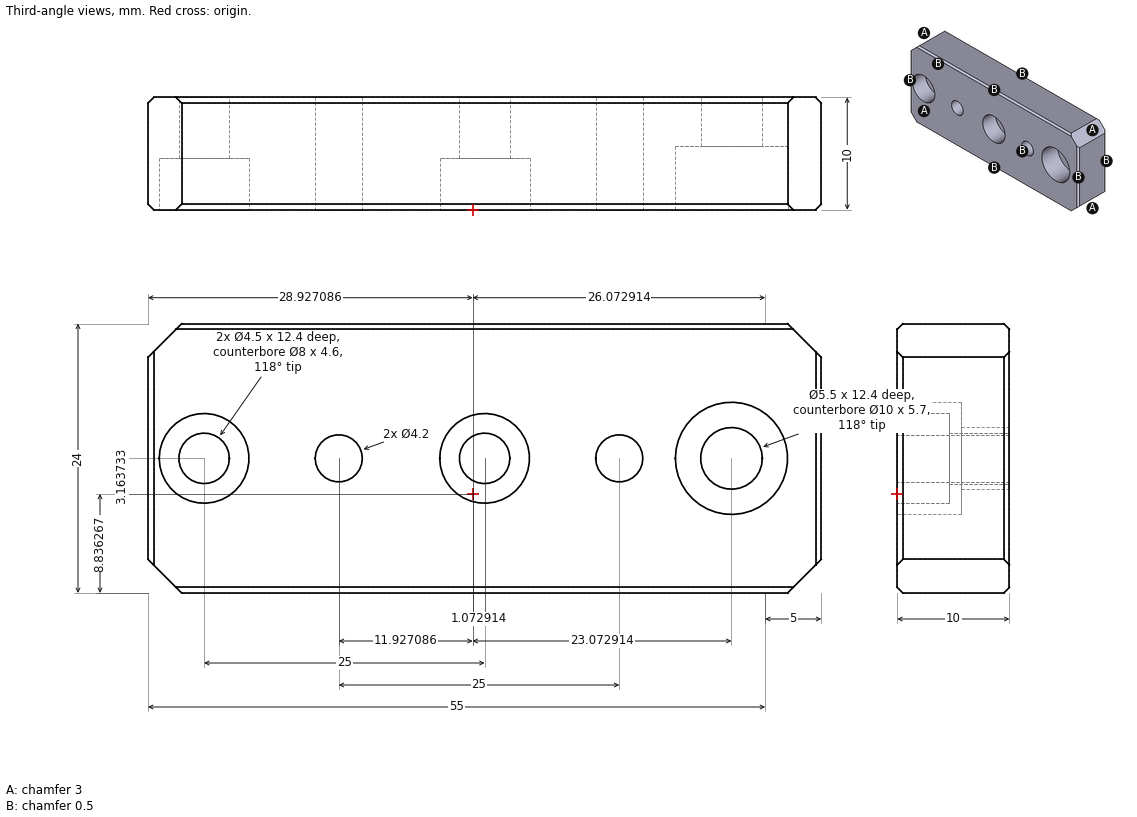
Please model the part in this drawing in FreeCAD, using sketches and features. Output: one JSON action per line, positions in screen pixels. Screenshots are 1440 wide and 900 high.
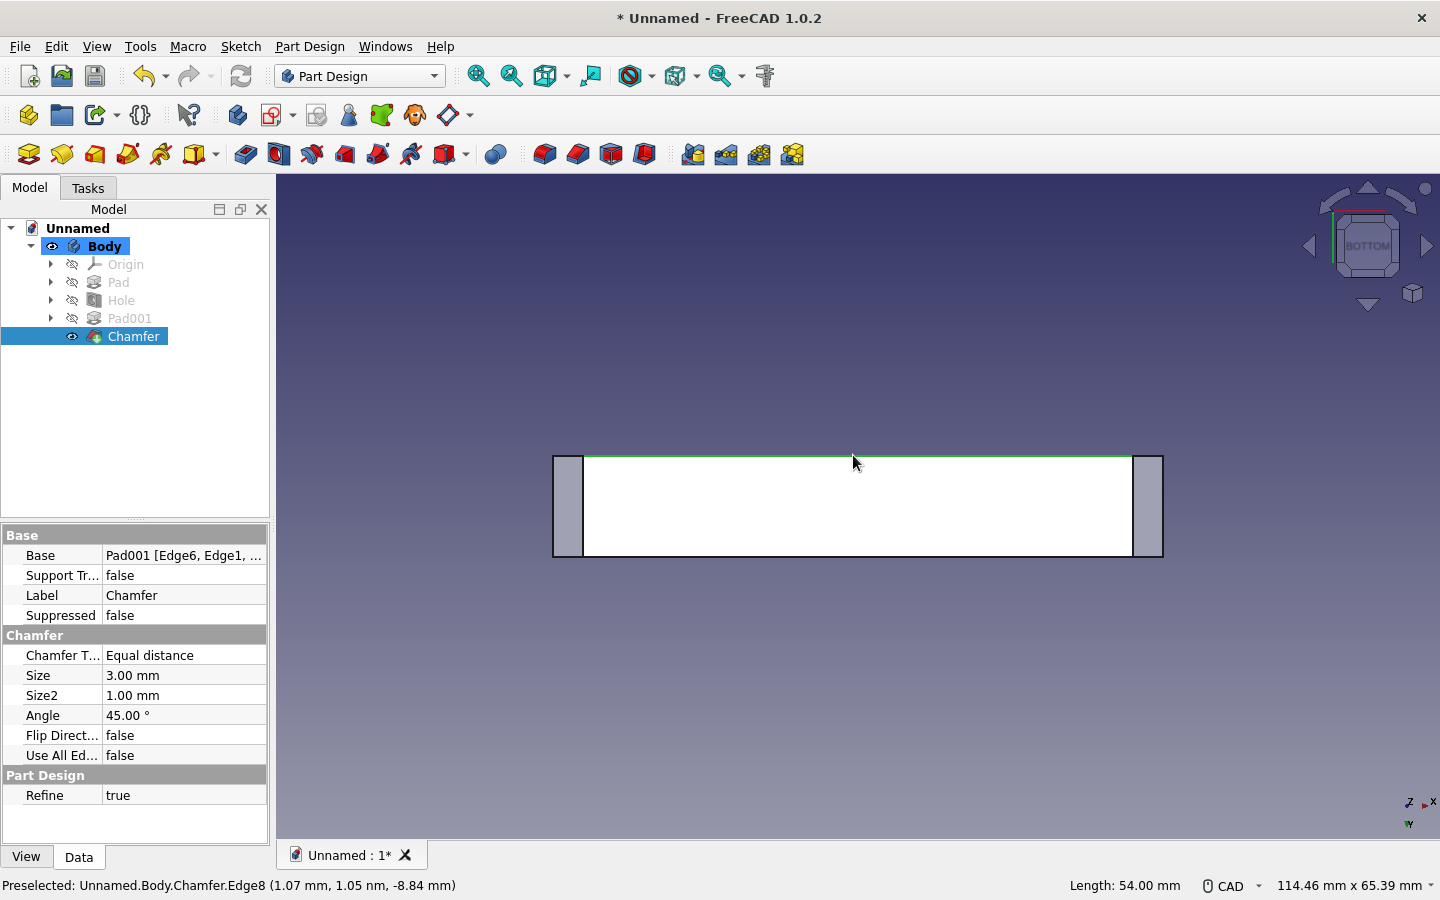
{"action": "key", "text": "0"}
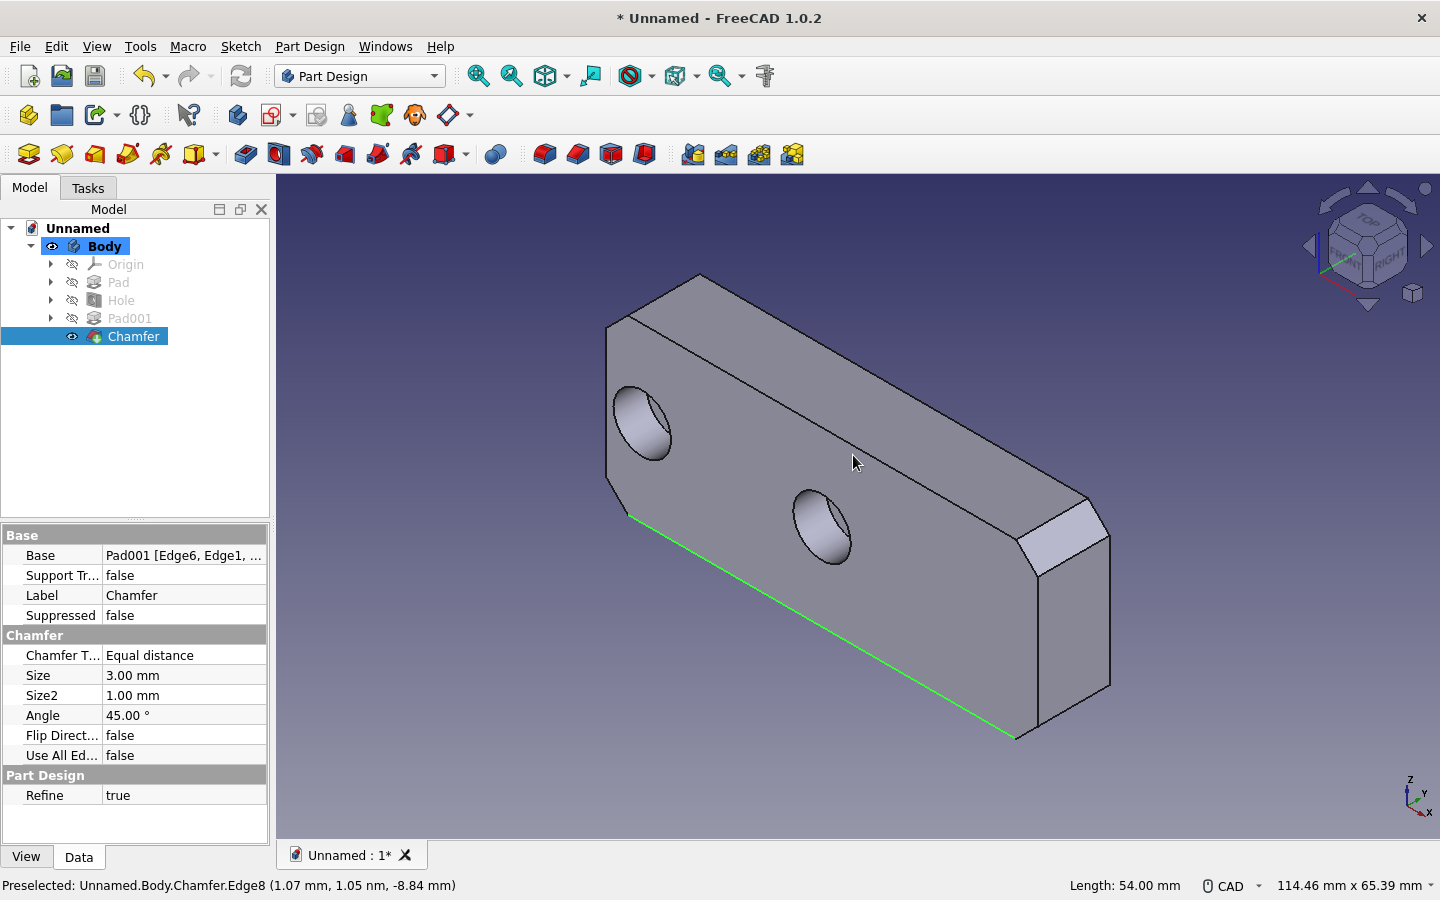
{"action": "left_click", "coordinate": [1038, 651], "text": "ctrl"}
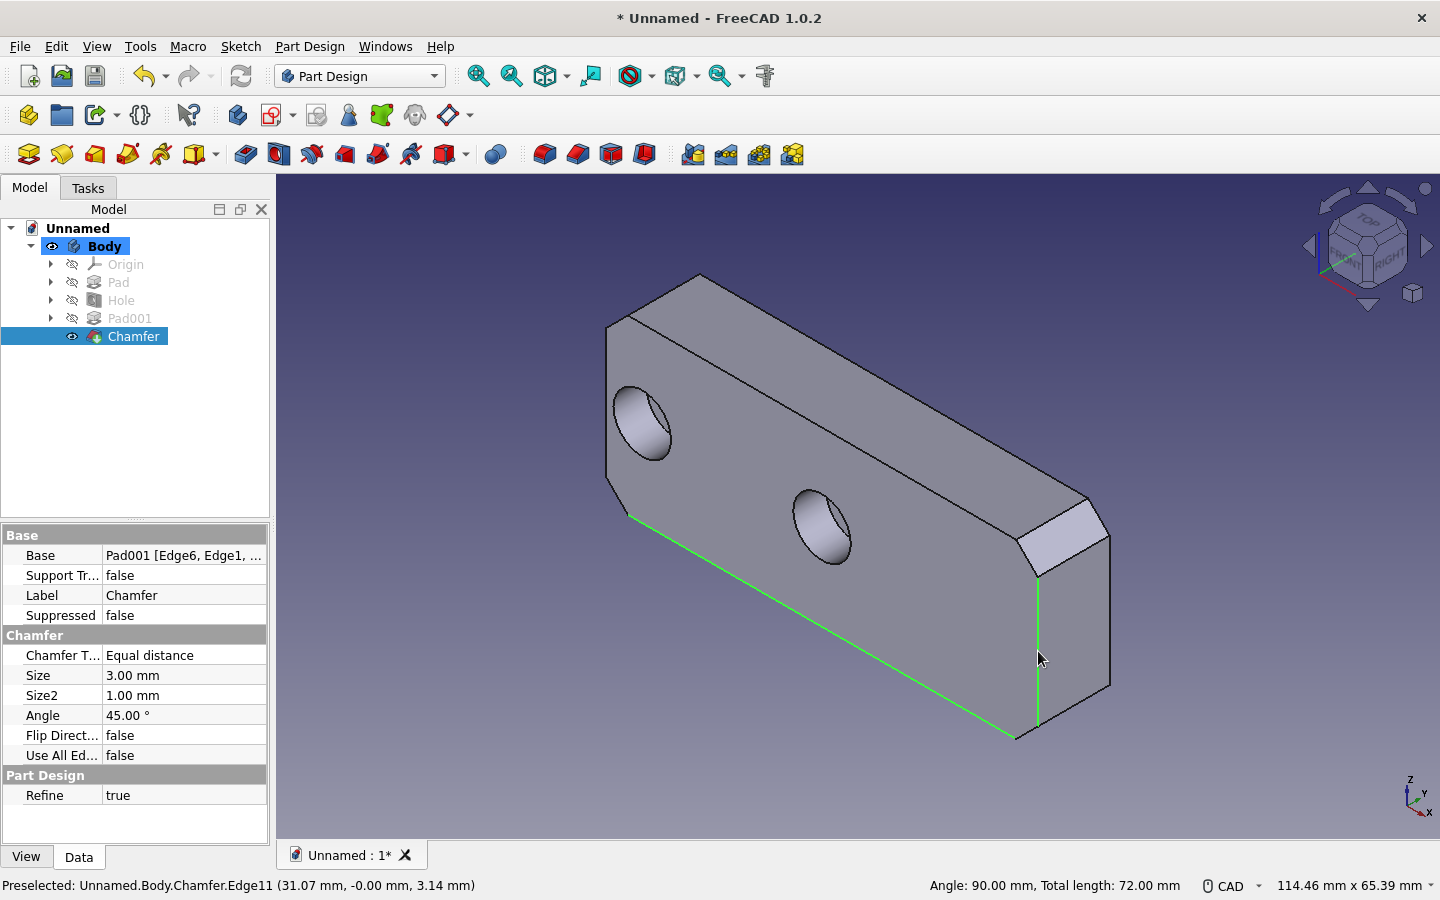
{"action": "left_click", "coordinate": [822, 427], "text": "ctrl"}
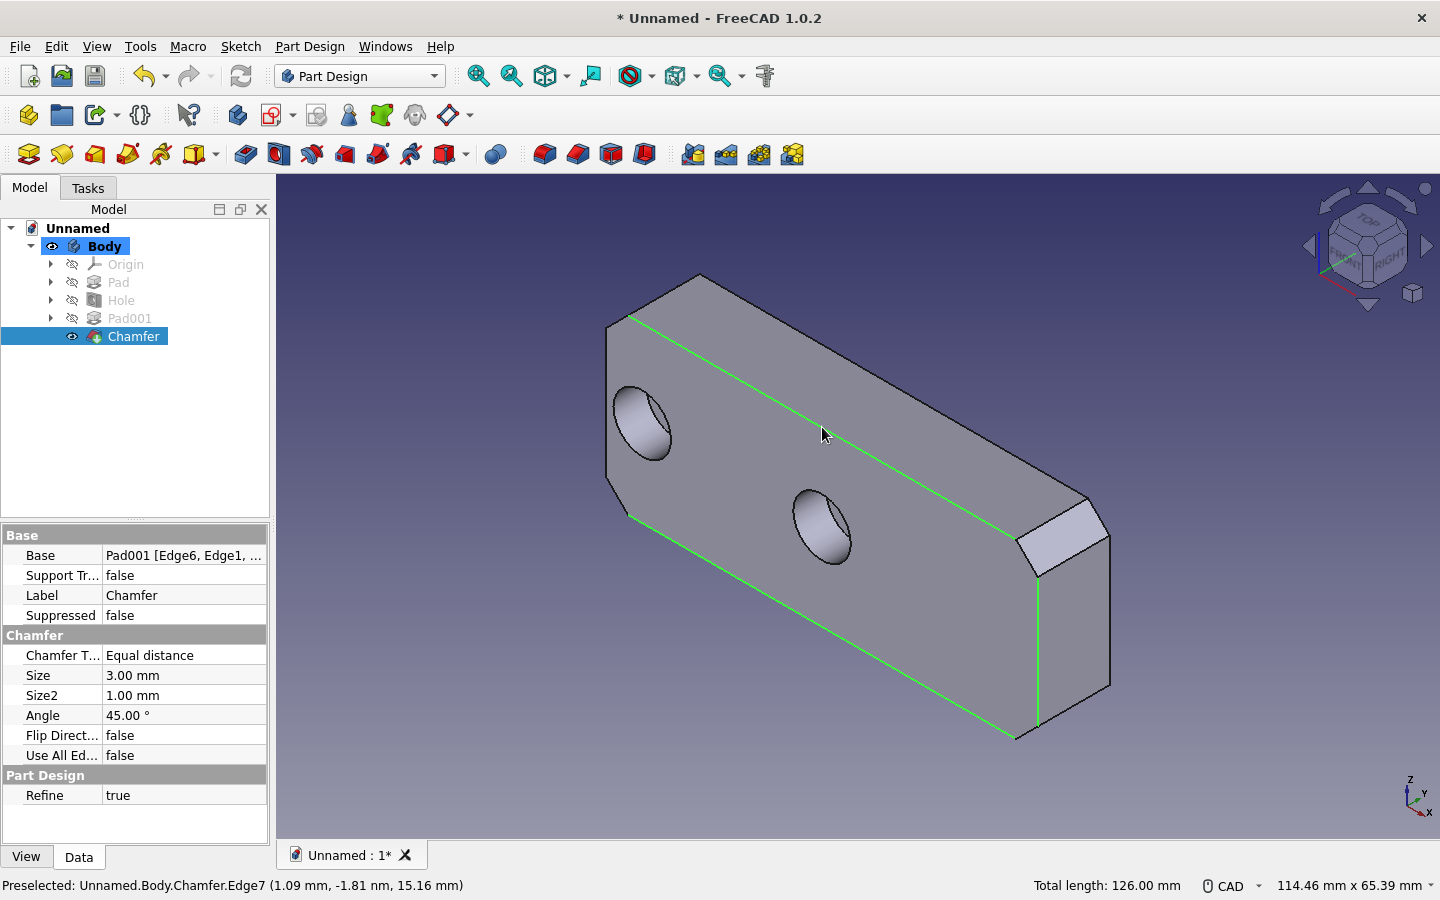
{"action": "key", "text": "2"}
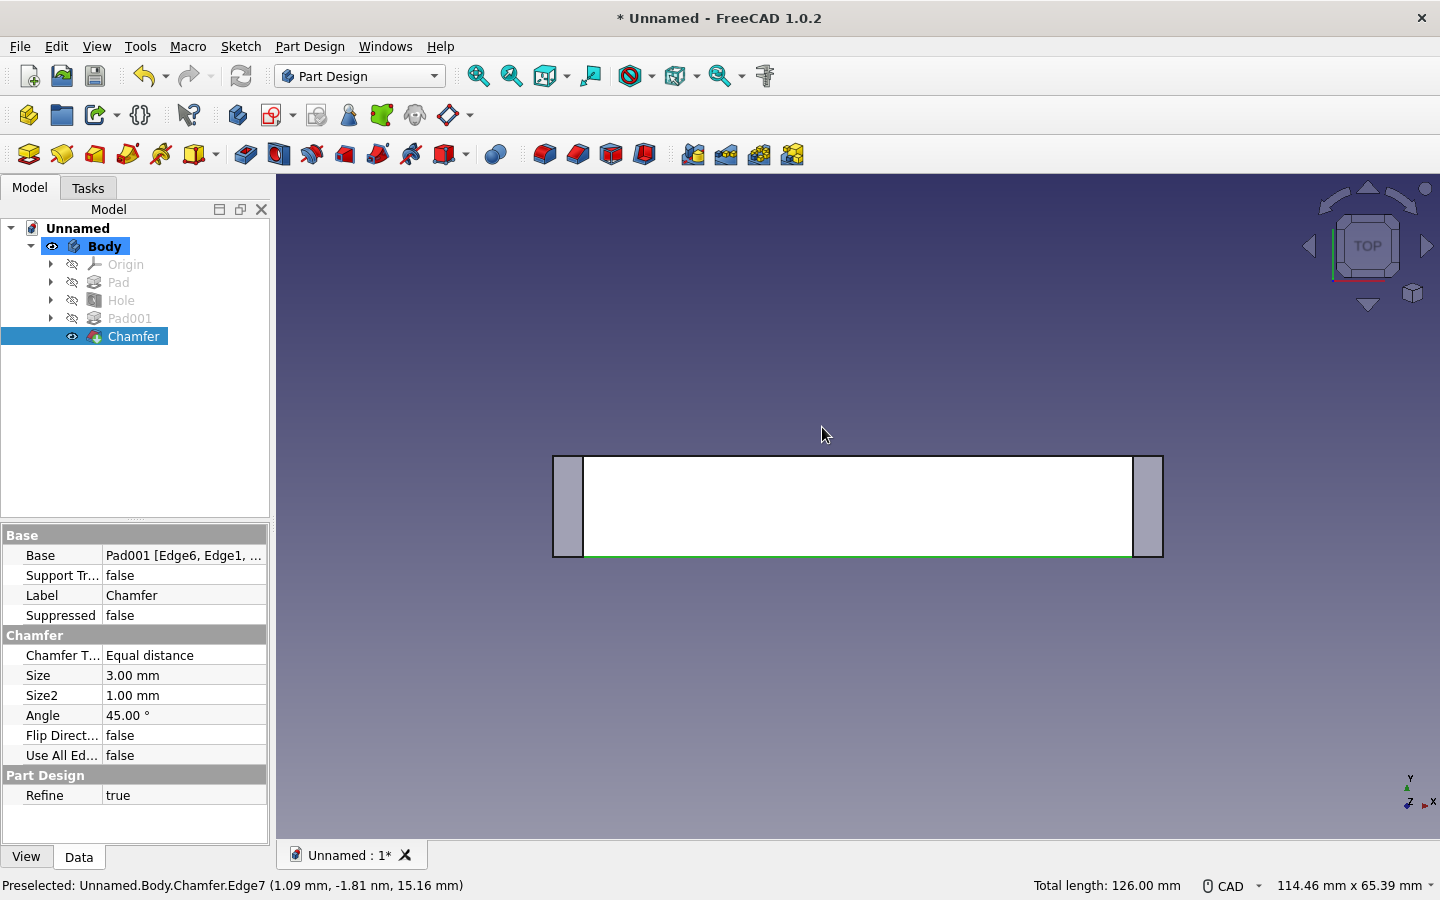
{"action": "left_click", "coordinate": [858, 455], "text": "ctrl"}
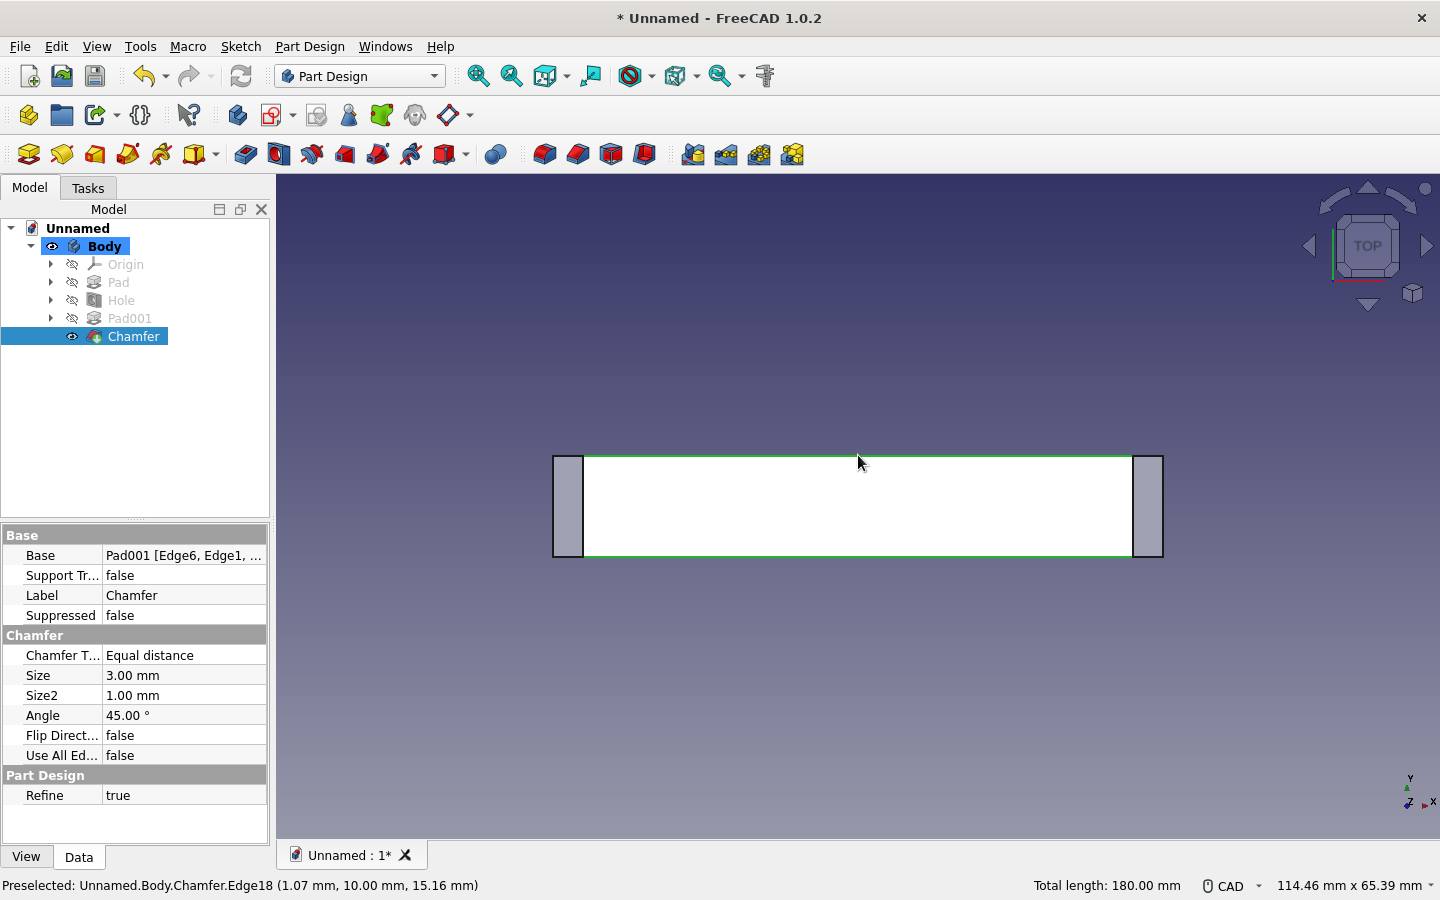
{"action": "key", "text": "1"}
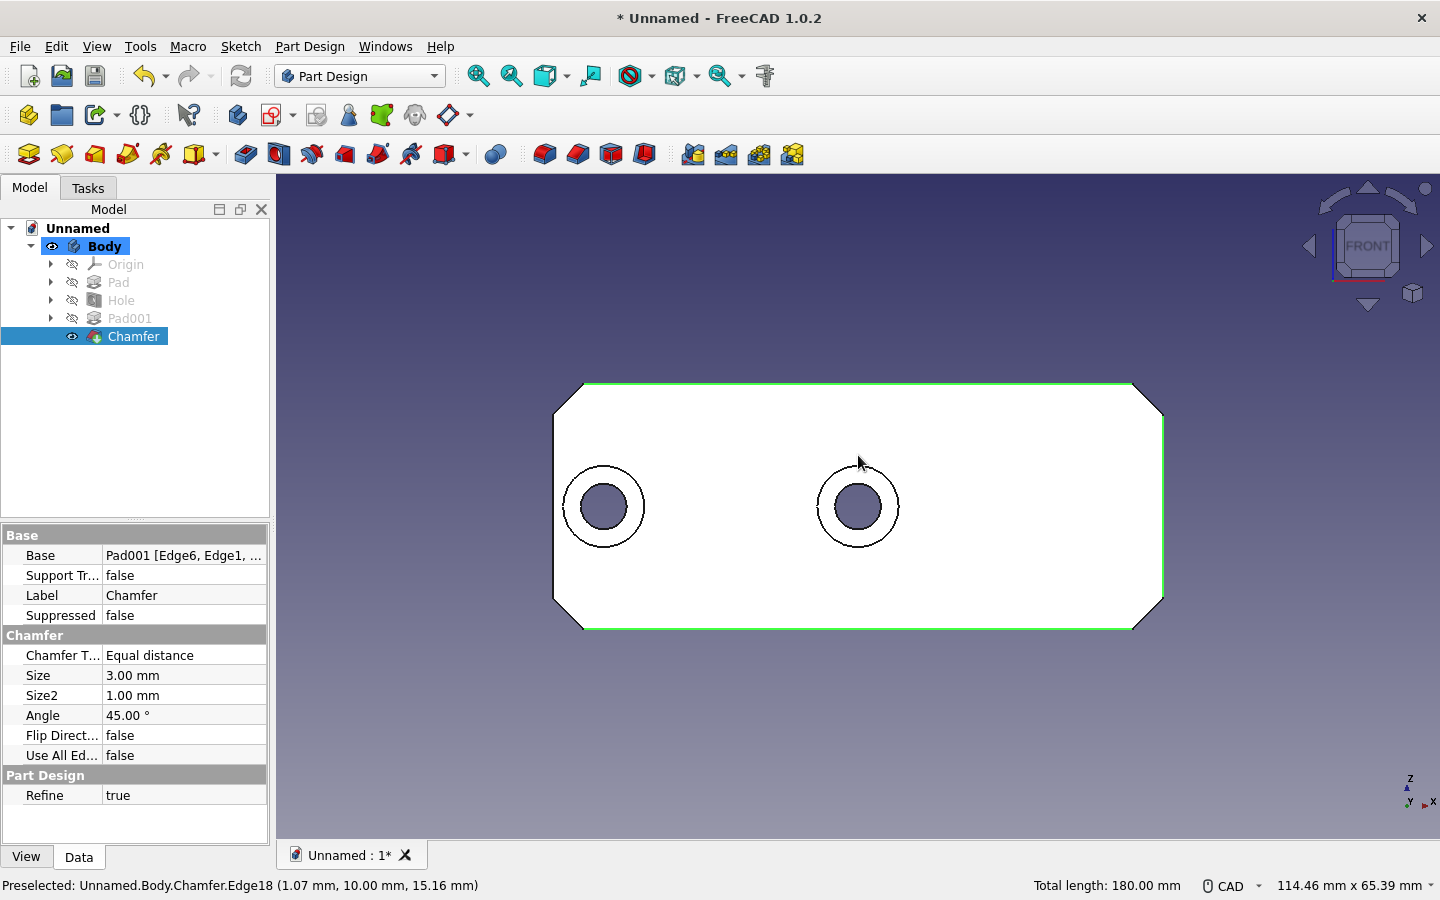
{"action": "key", "text": "3"}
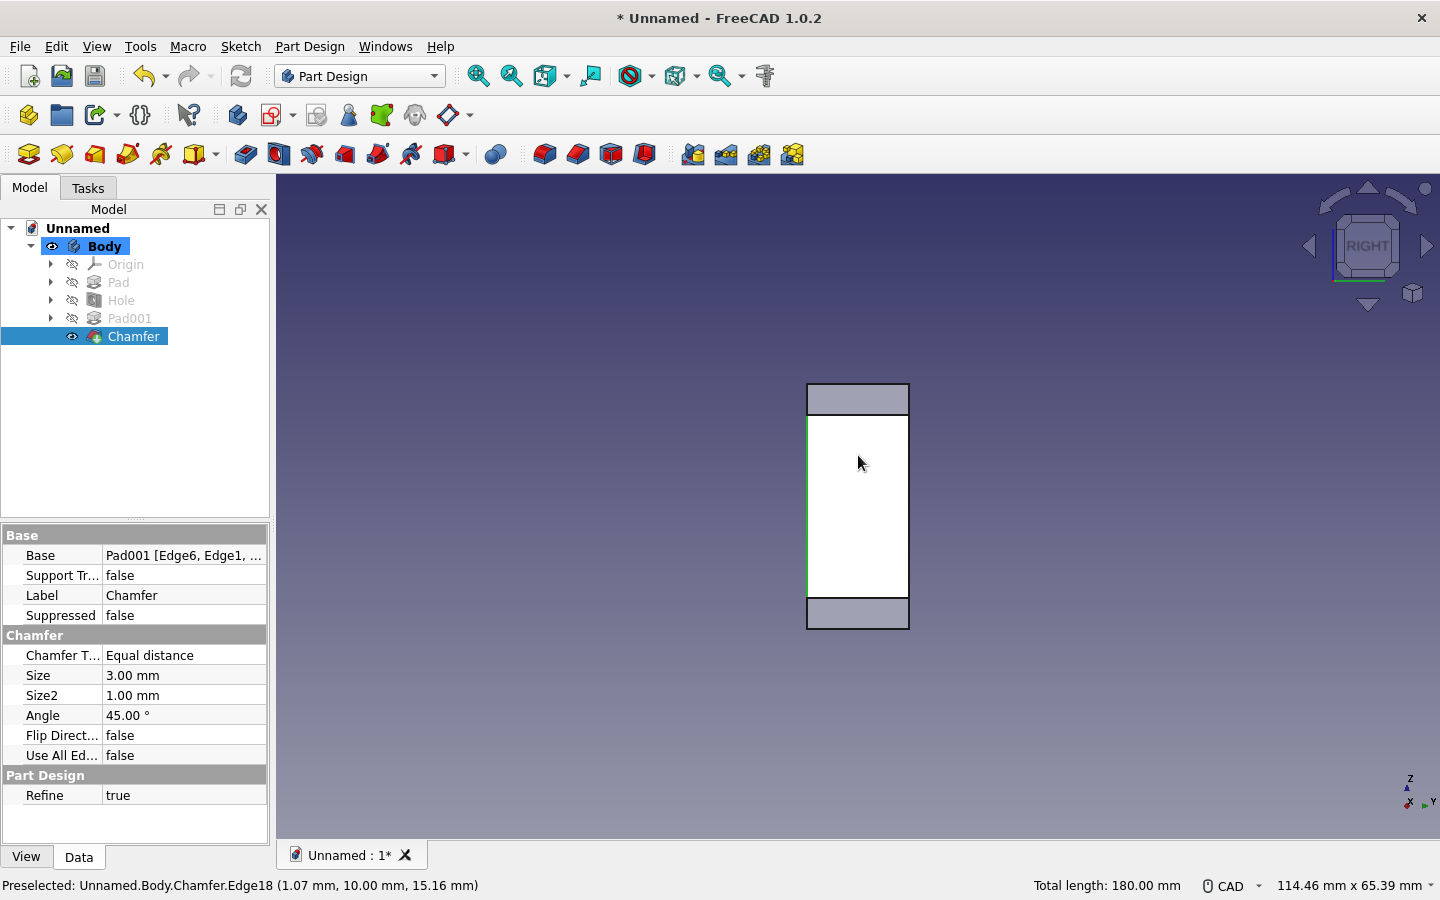
{"action": "key", "text": "v f"}